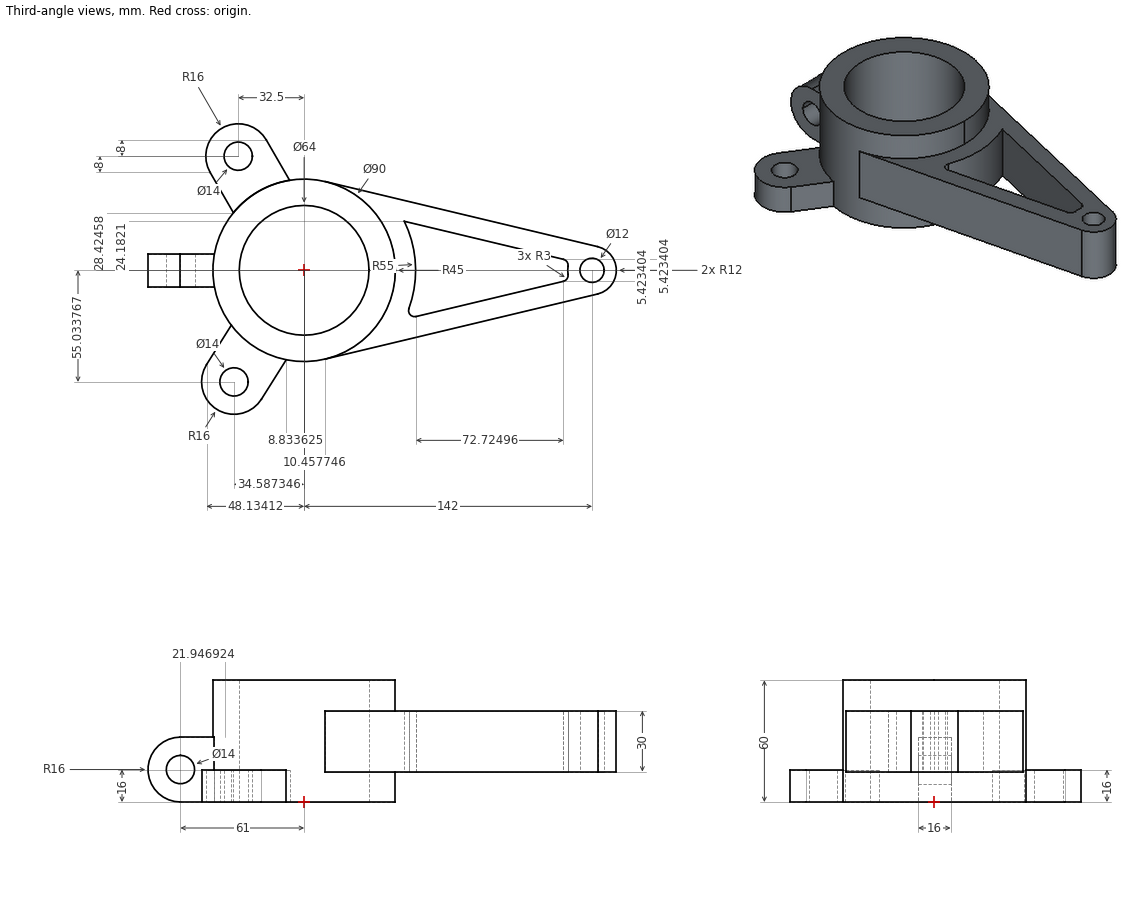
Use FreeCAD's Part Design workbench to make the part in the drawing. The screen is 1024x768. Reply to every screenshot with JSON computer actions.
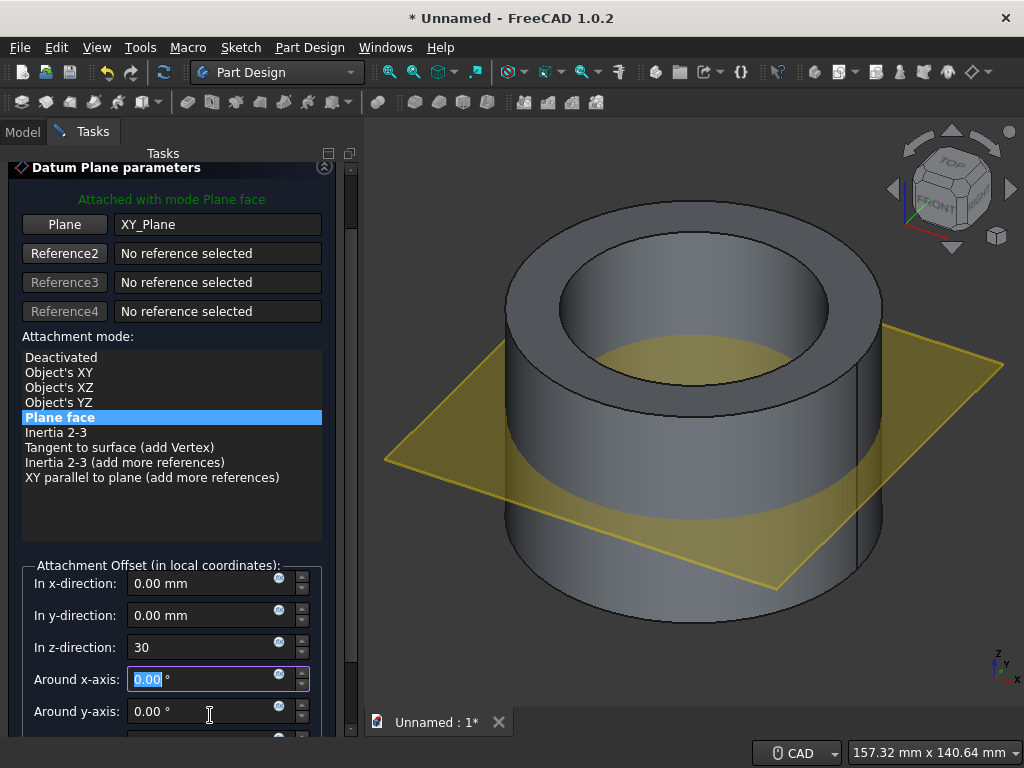
{"action": "scroll", "coordinate": [351, 450], "scroll_direction": "up", "scroll_amount": 2}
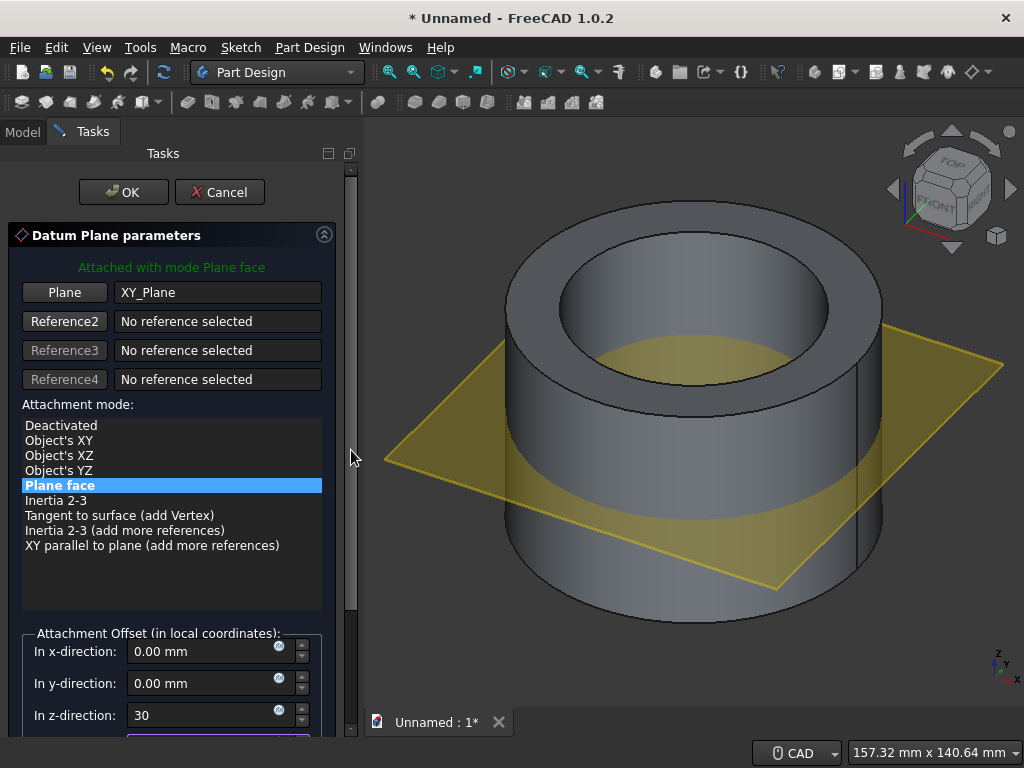
{"action": "left_click", "coordinate": [124, 192]}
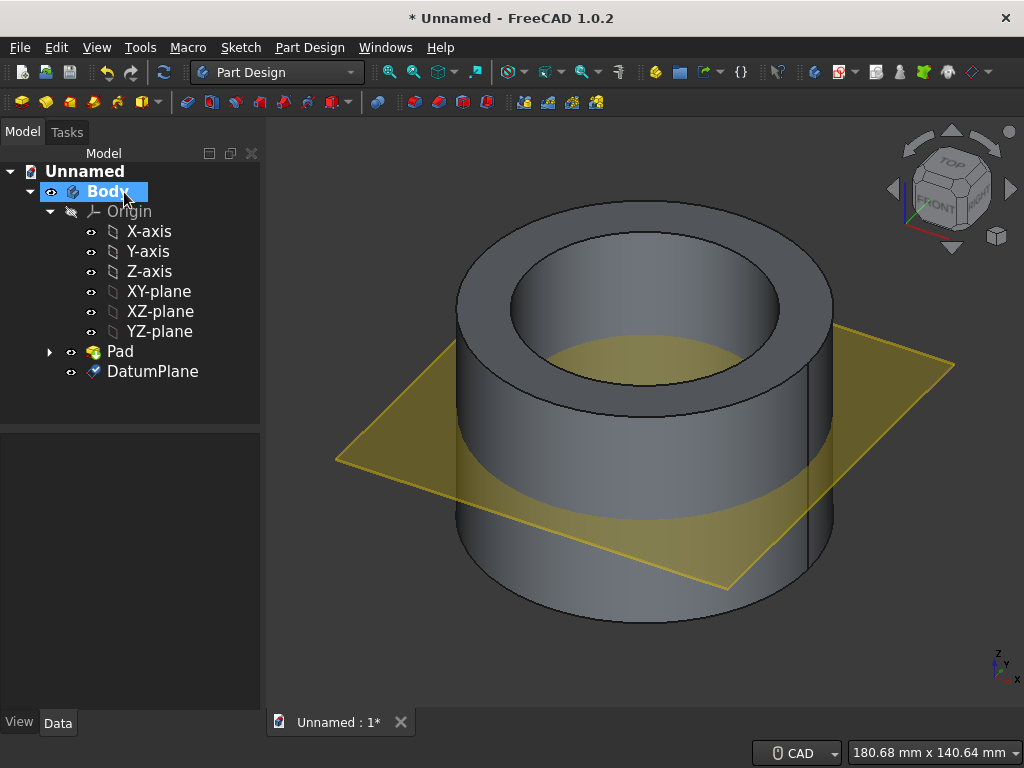
{"action": "left_click", "coordinate": [116, 372]}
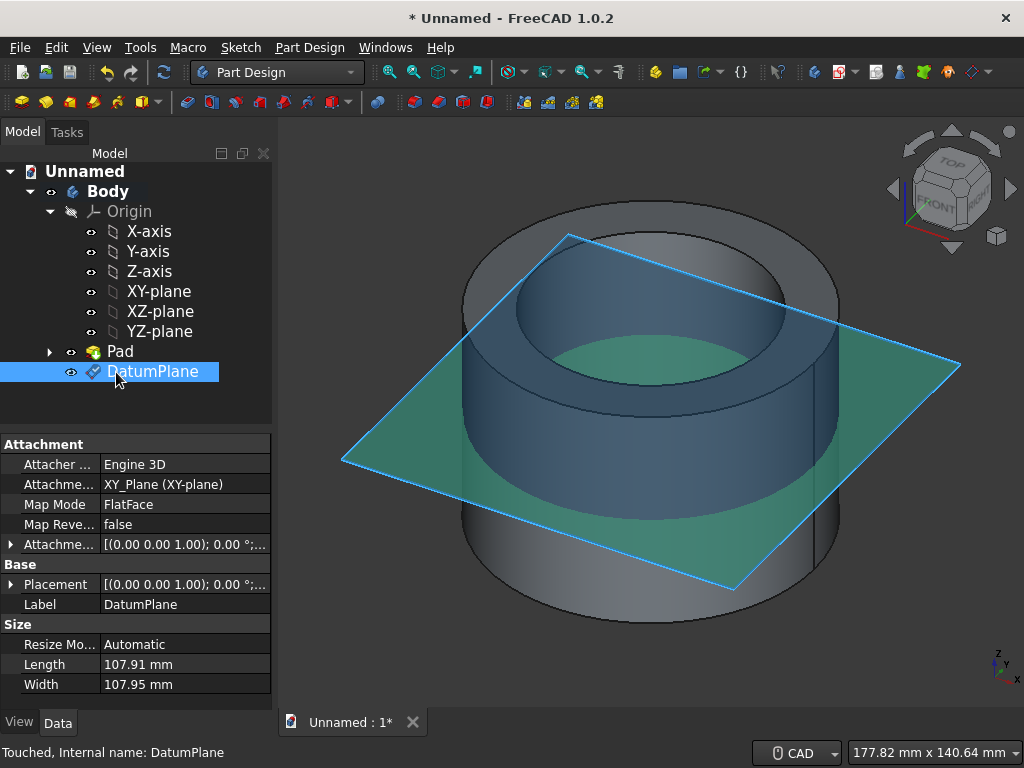
{"action": "left_click", "coordinate": [840, 72]}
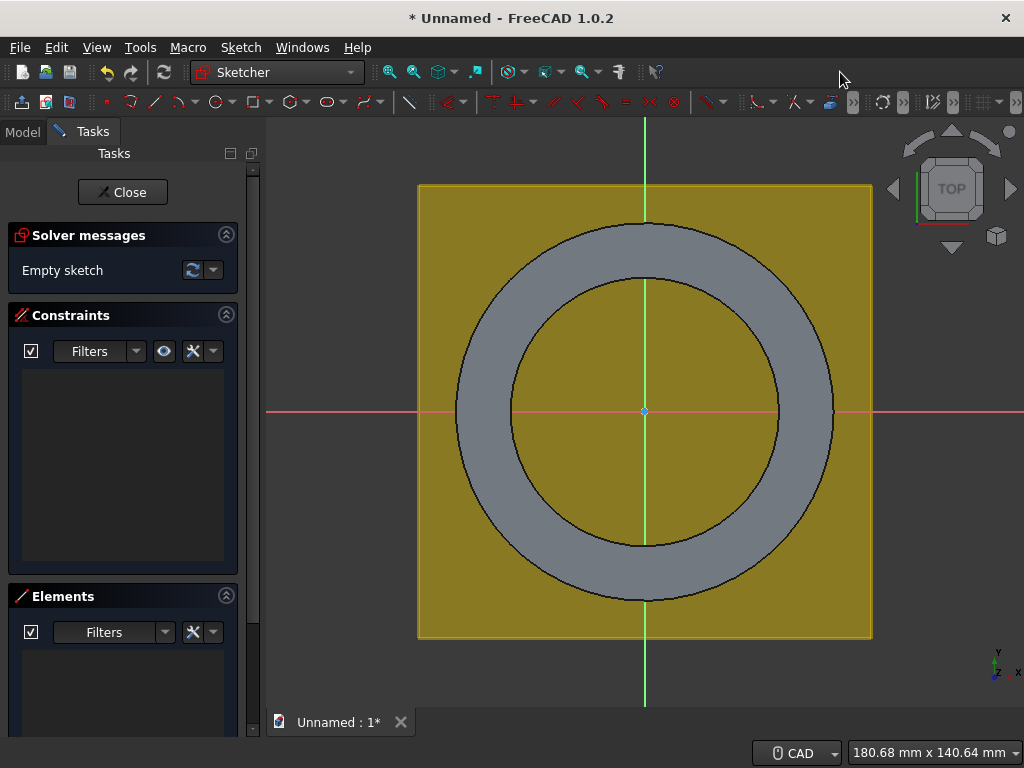
{"action": "left_click", "coordinate": [70, 102]}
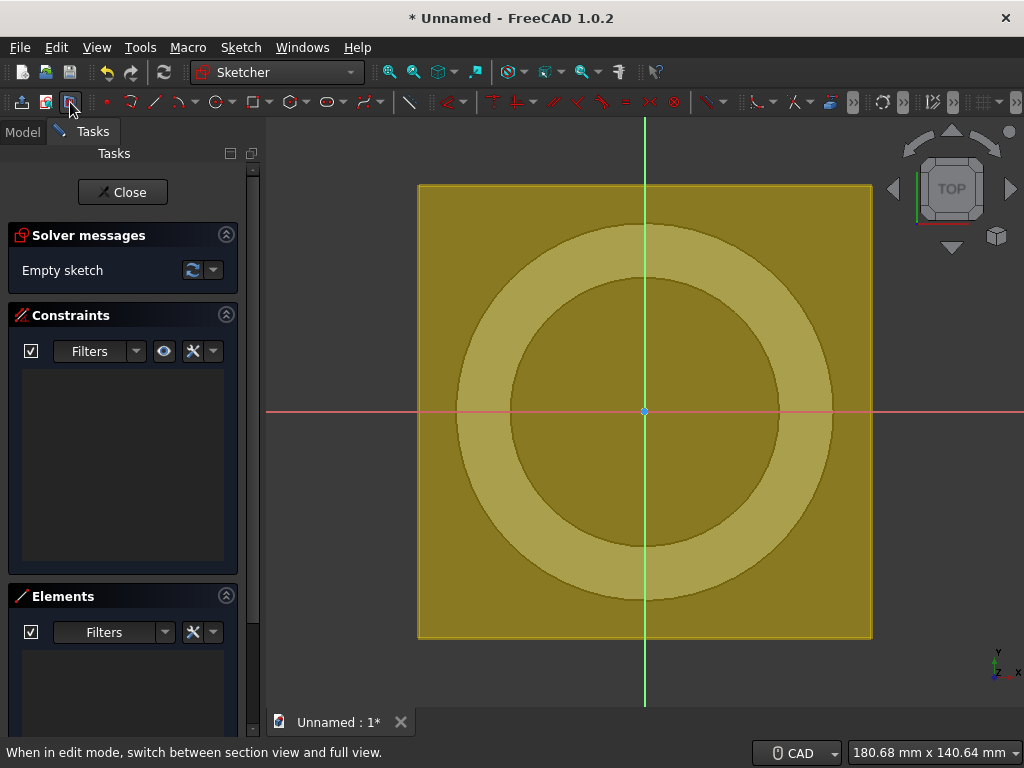
{"action": "scroll", "coordinate": [294, 412], "scroll_direction": "down", "scroll_amount": 4}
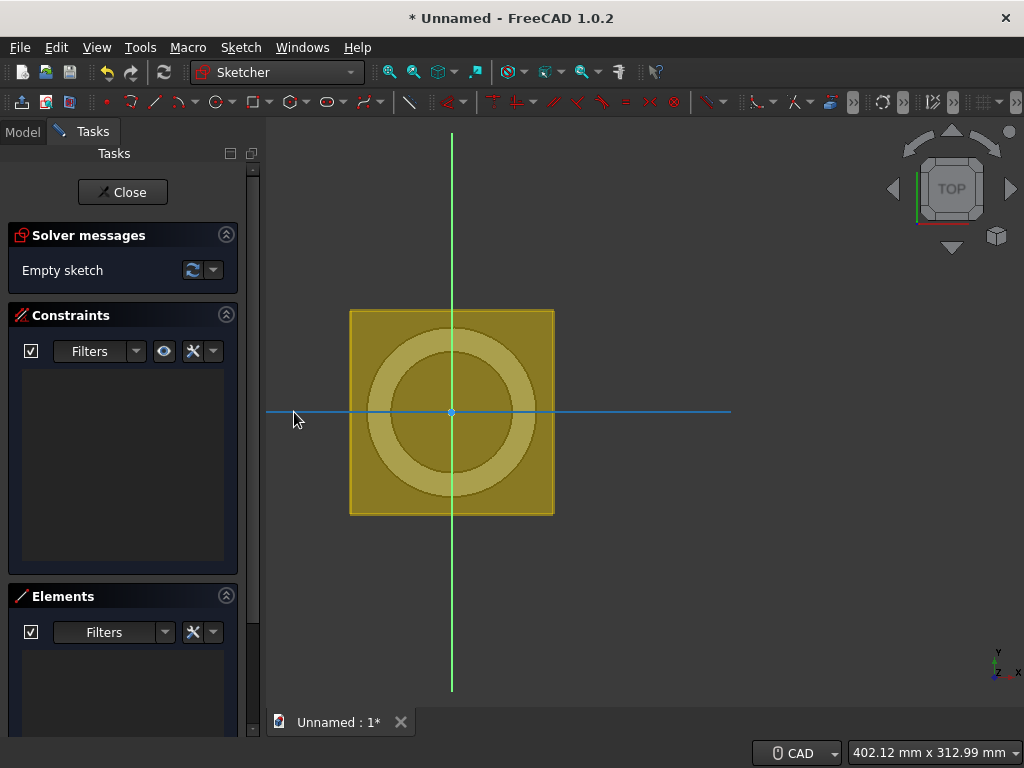
{"action": "scroll", "coordinate": [638, 413], "scroll_direction": "up", "scroll_amount": 2}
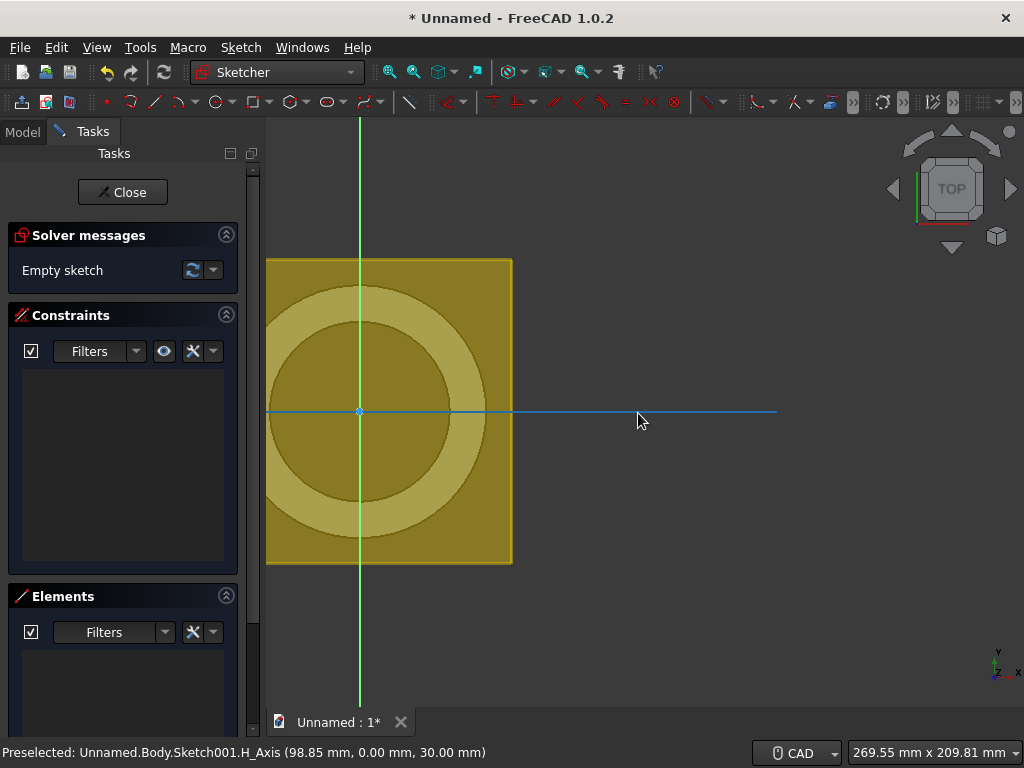
{"action": "left_click", "coordinate": [156, 102]}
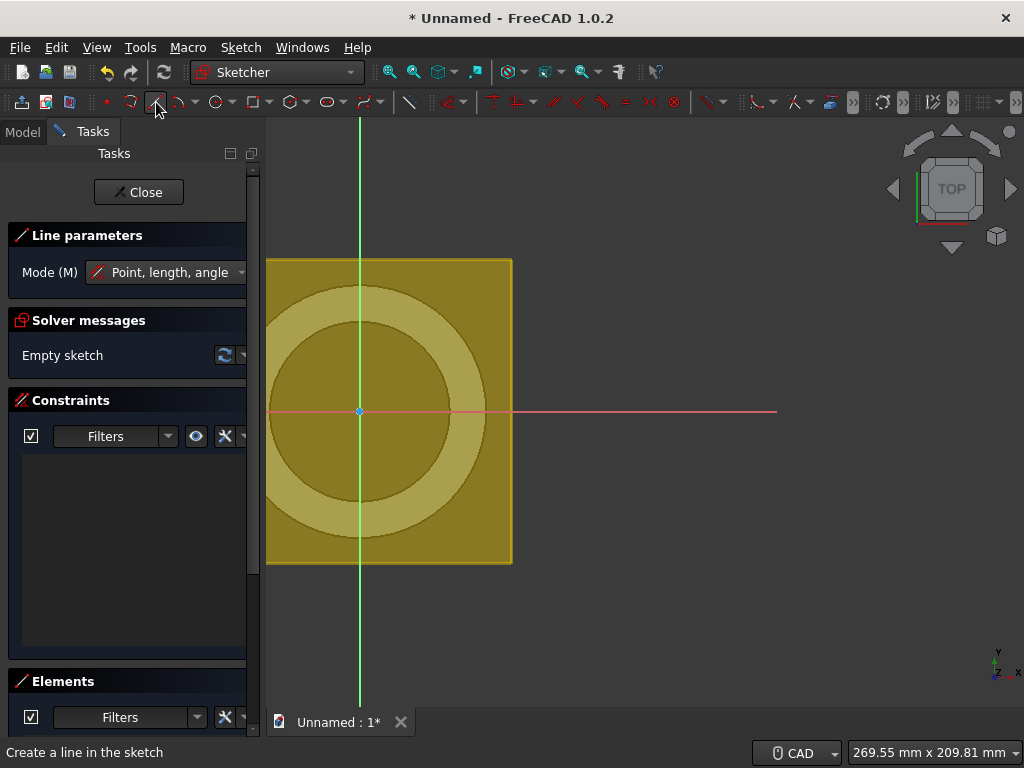
{"action": "left_click", "coordinate": [389, 535]}
{"action": "left_click", "coordinate": [767, 444]}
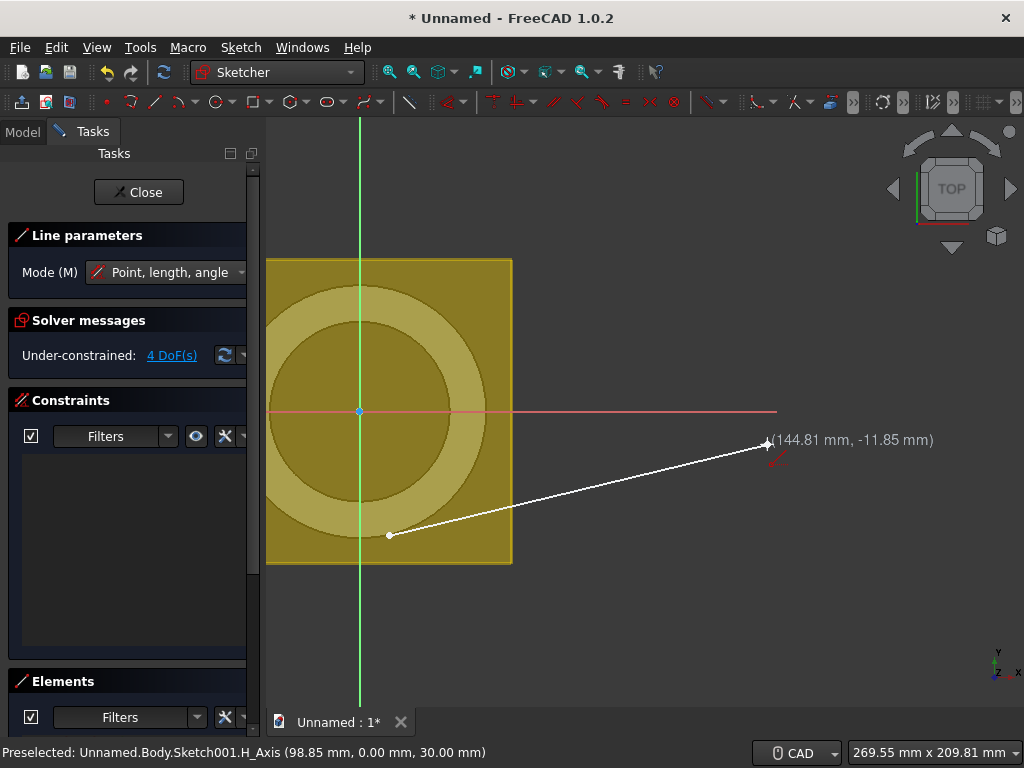
{"action": "left_click", "coordinate": [767, 379]}
{"action": "left_click", "coordinate": [389, 289]}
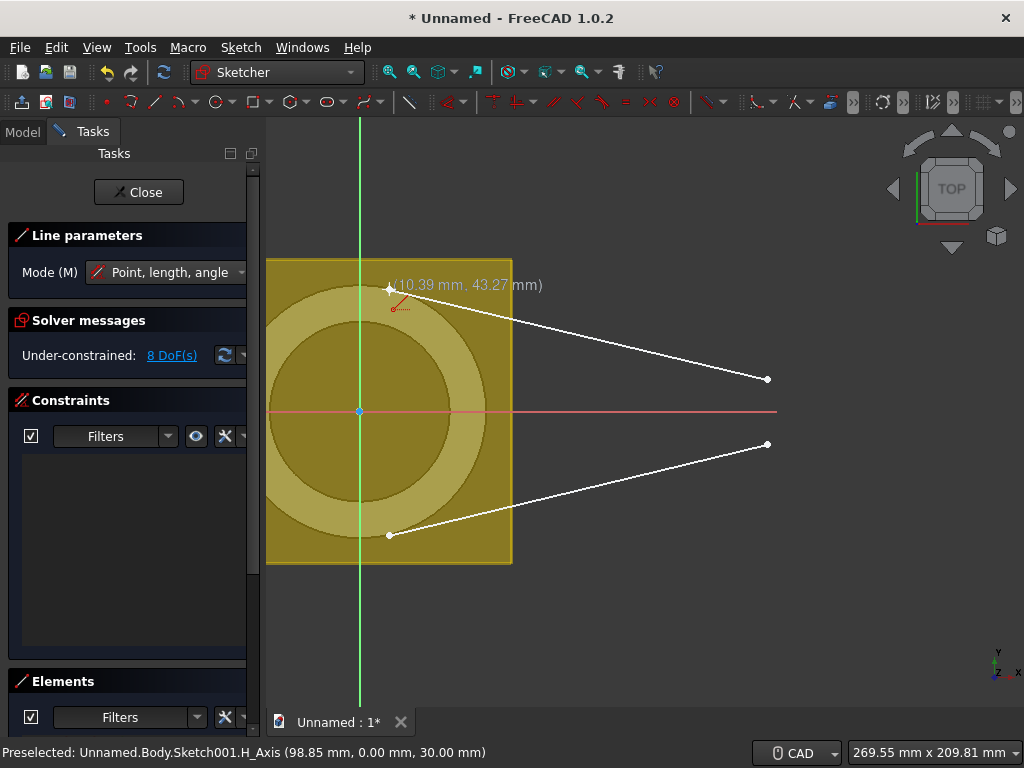
{"action": "key", "text": "g 3 a"}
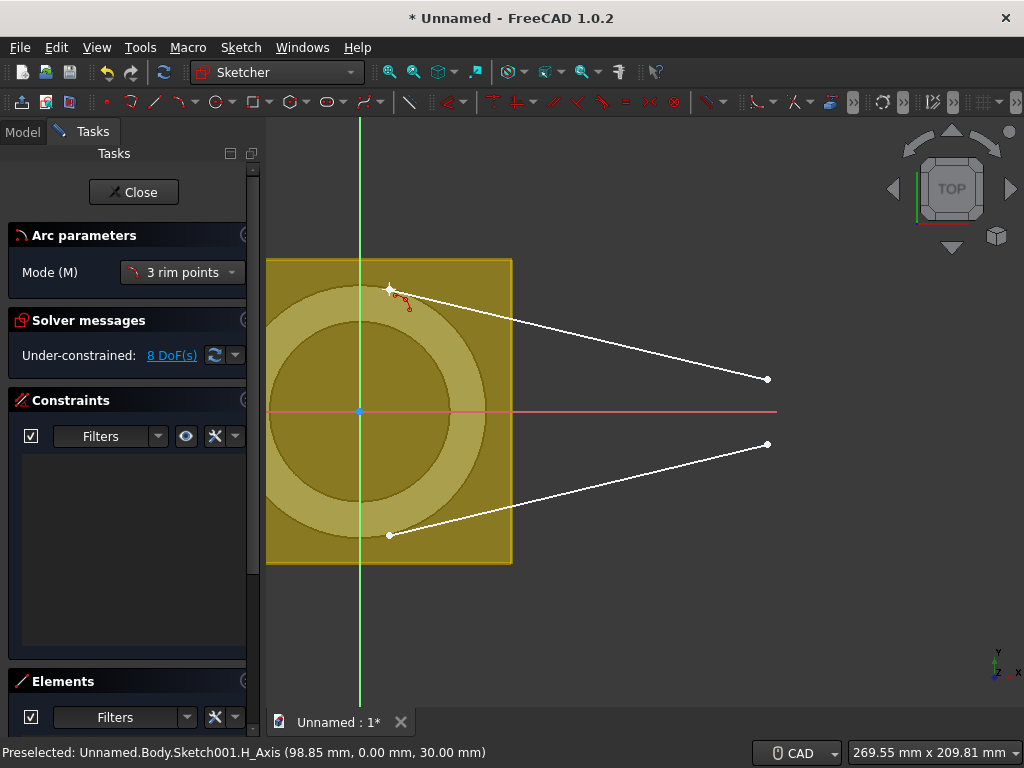
{"action": "left_click", "coordinate": [767, 445]}
{"action": "left_click", "coordinate": [767, 380]}
{"action": "left_click", "coordinate": [788, 429]}